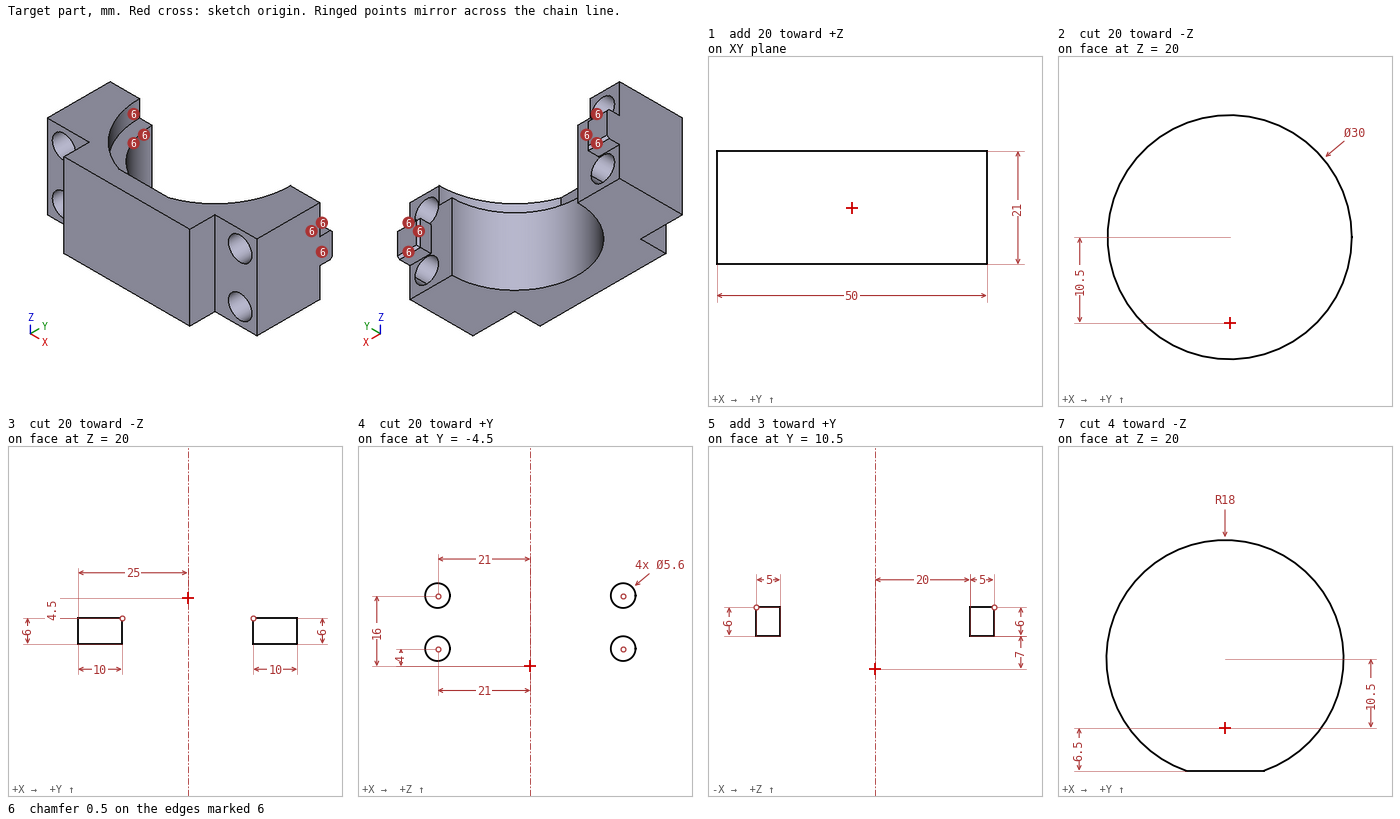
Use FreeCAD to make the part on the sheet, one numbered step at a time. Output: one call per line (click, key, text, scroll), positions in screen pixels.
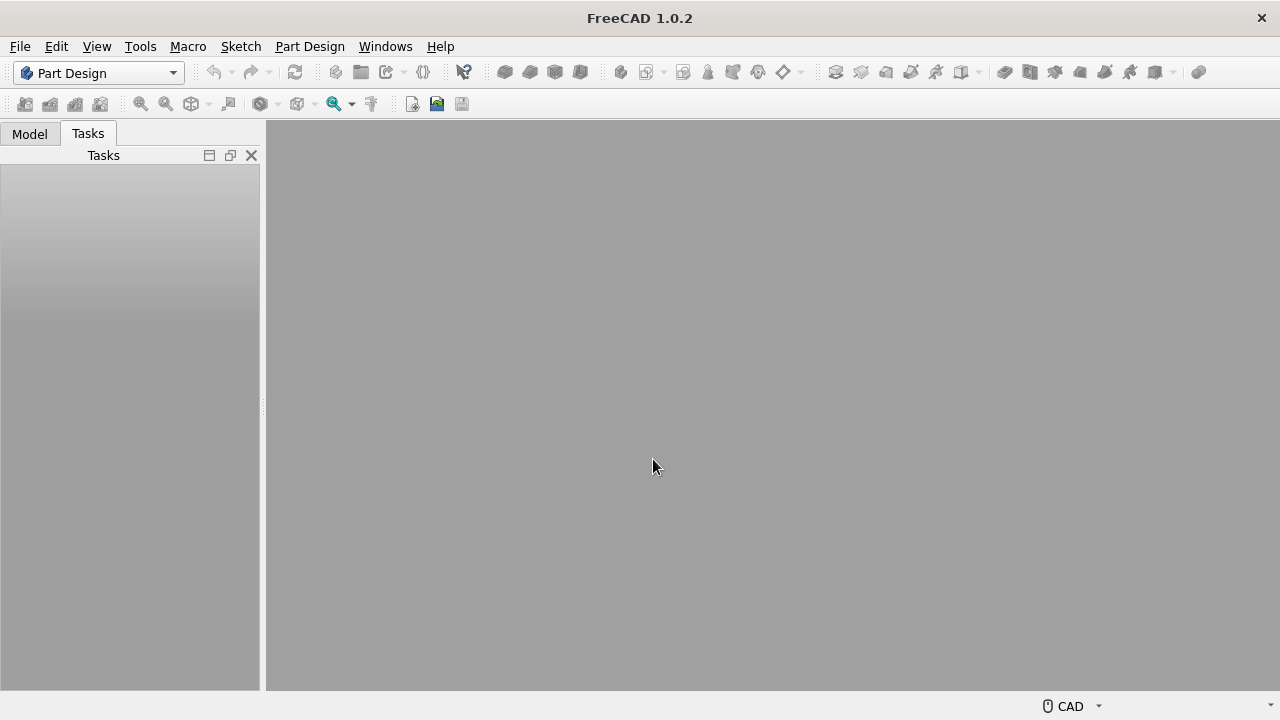
key(ctrl+n)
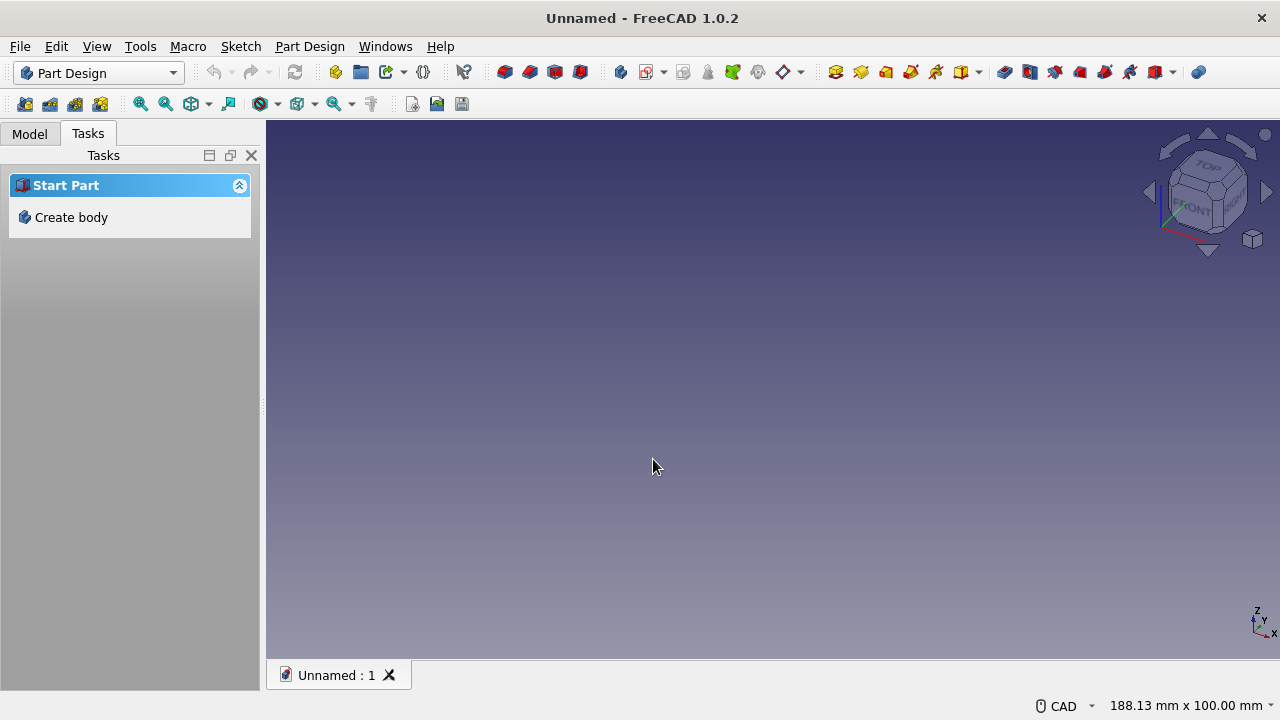
click(646, 72)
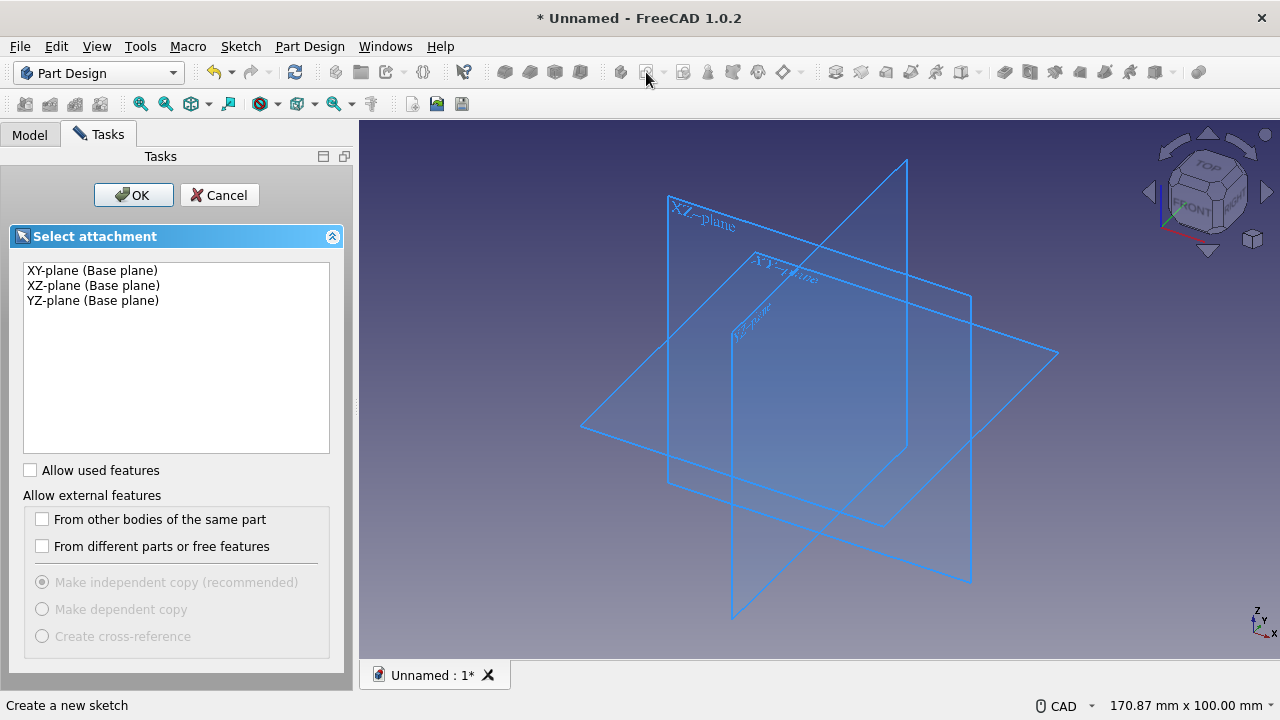
click(84, 270)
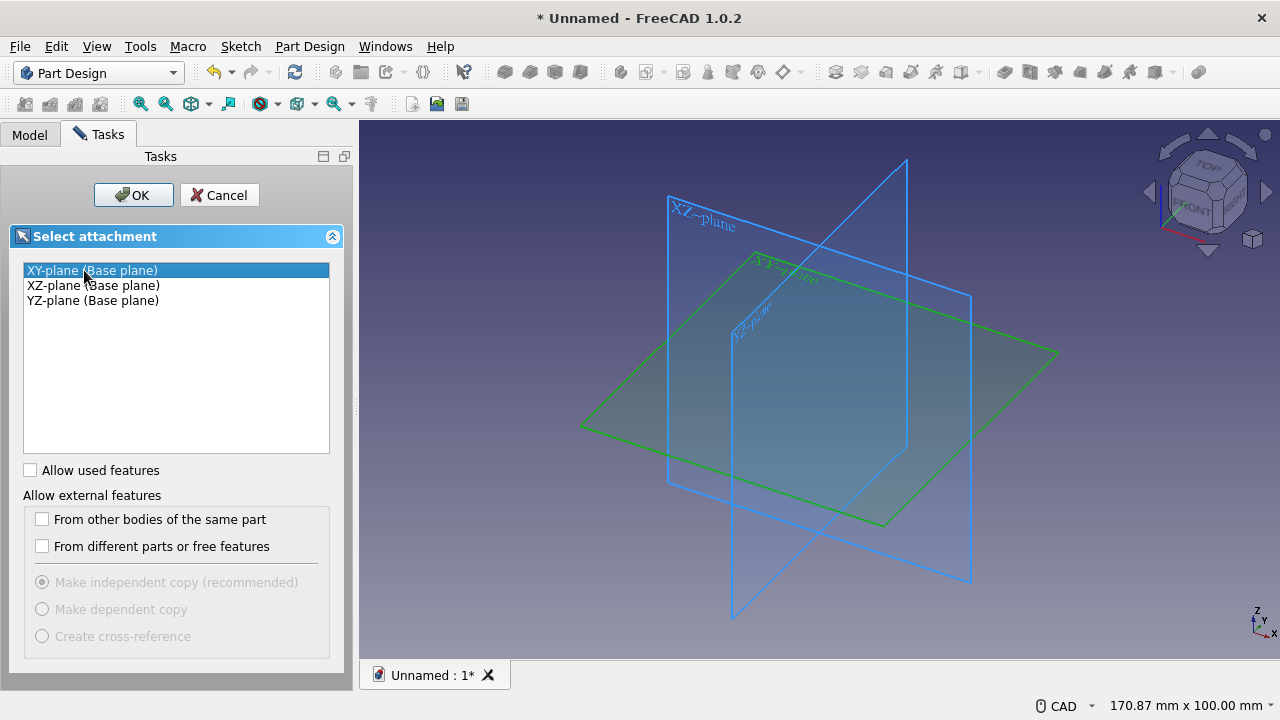
click(134, 195)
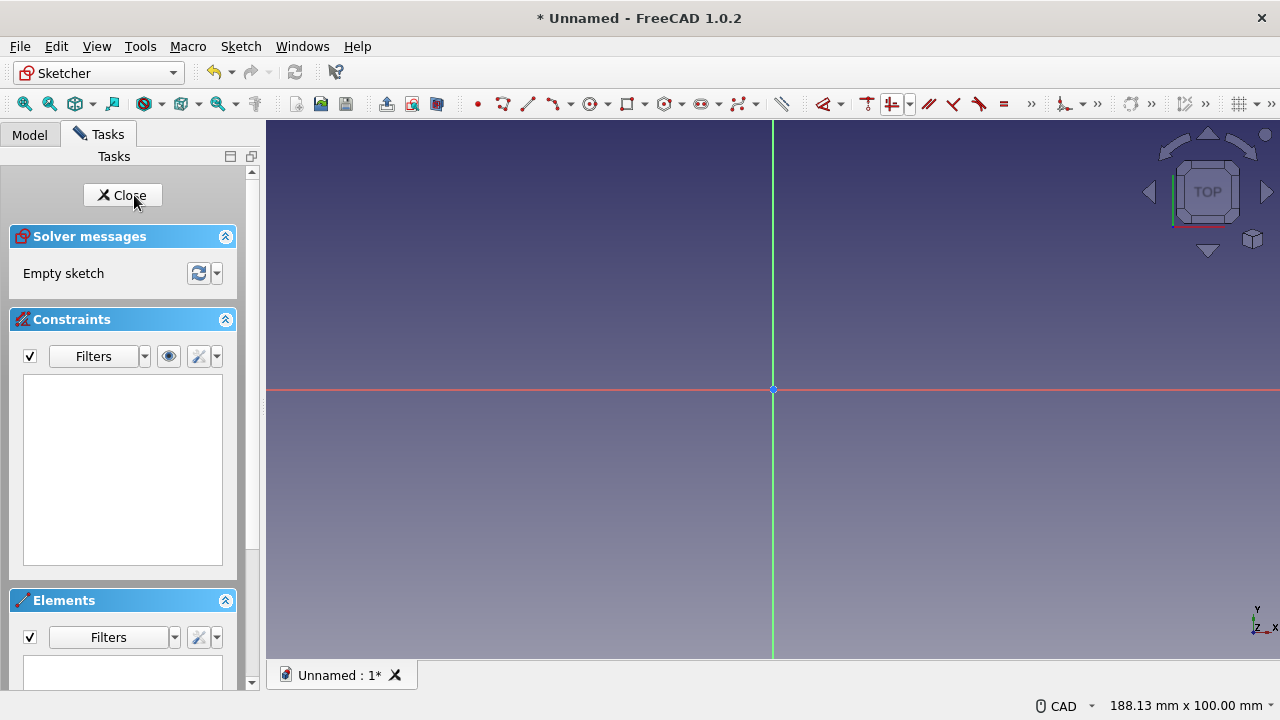
scroll(829, 390, up, 4)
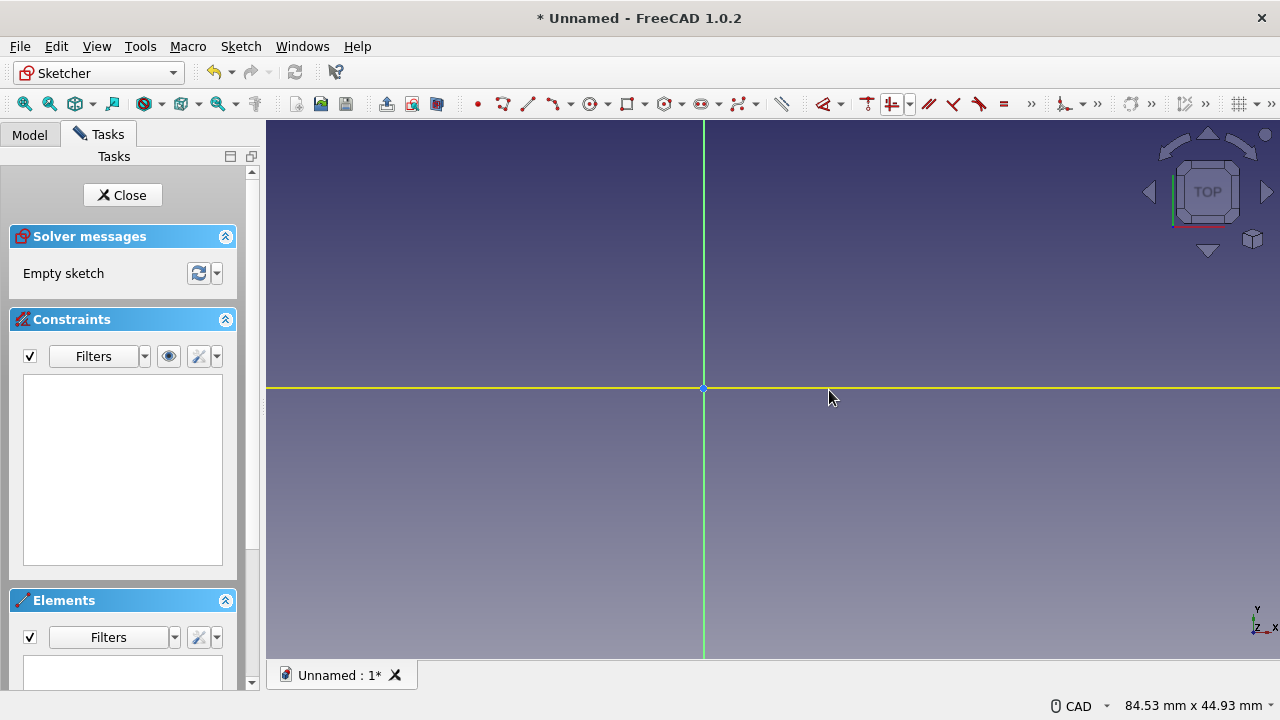
key(g)
key(v)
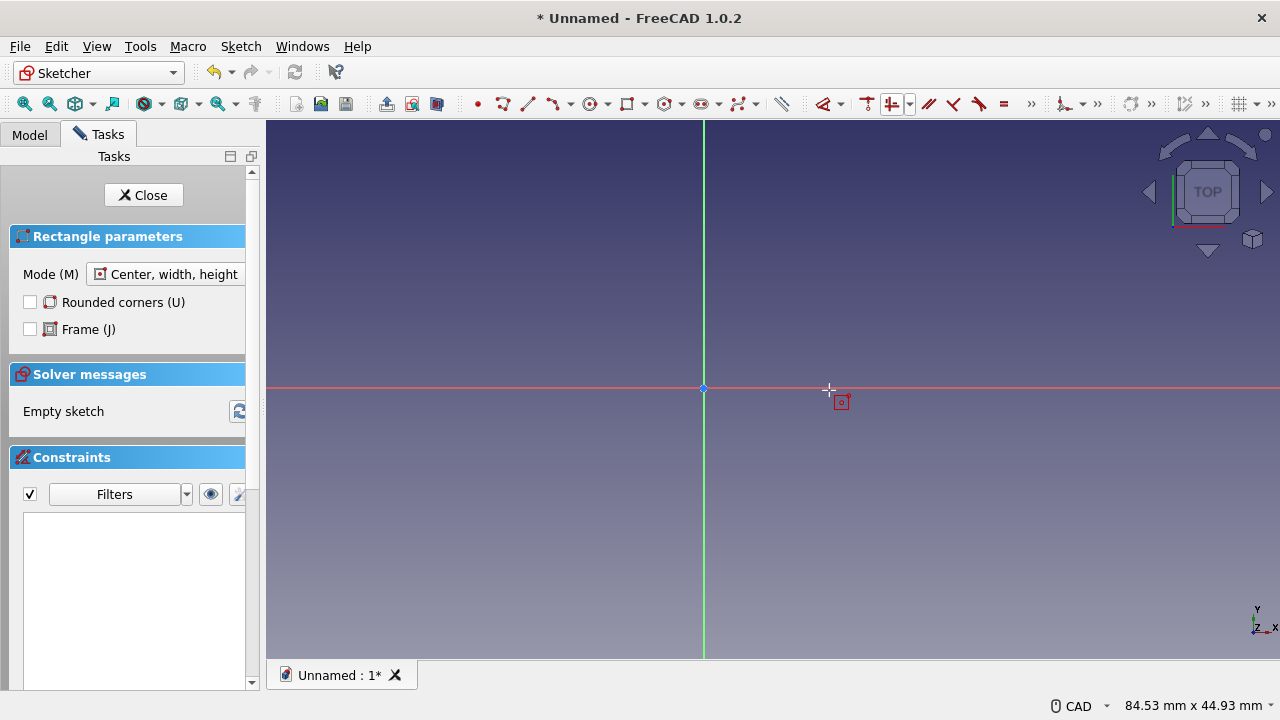
click(704, 388)
move(1004, 262)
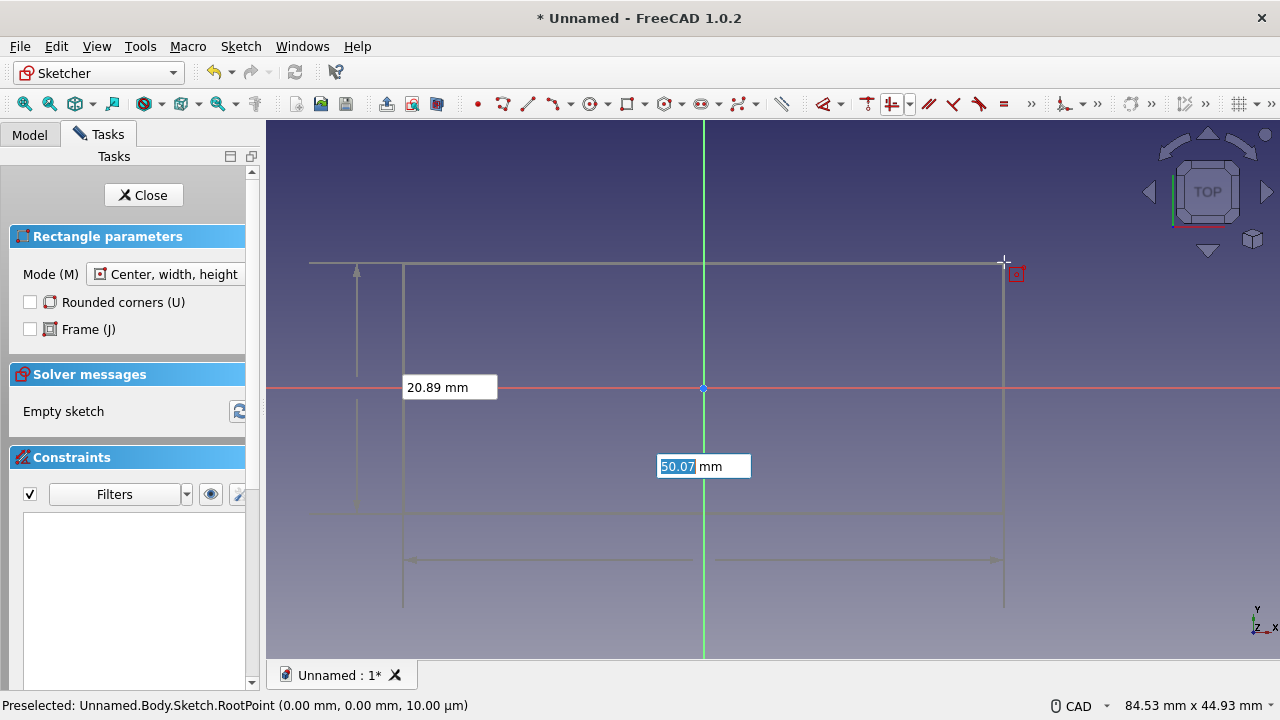
text(50)
key(Tab)
text(21)
key(Return)
key(Escape)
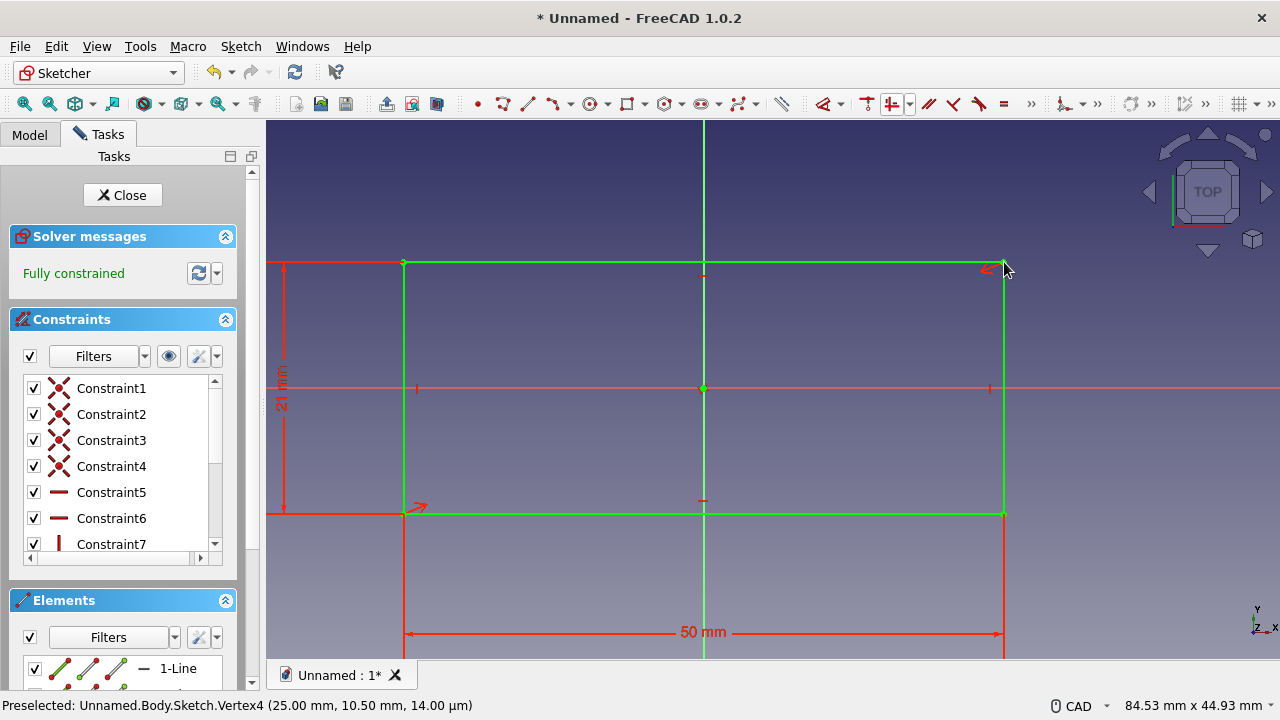
click(123, 195)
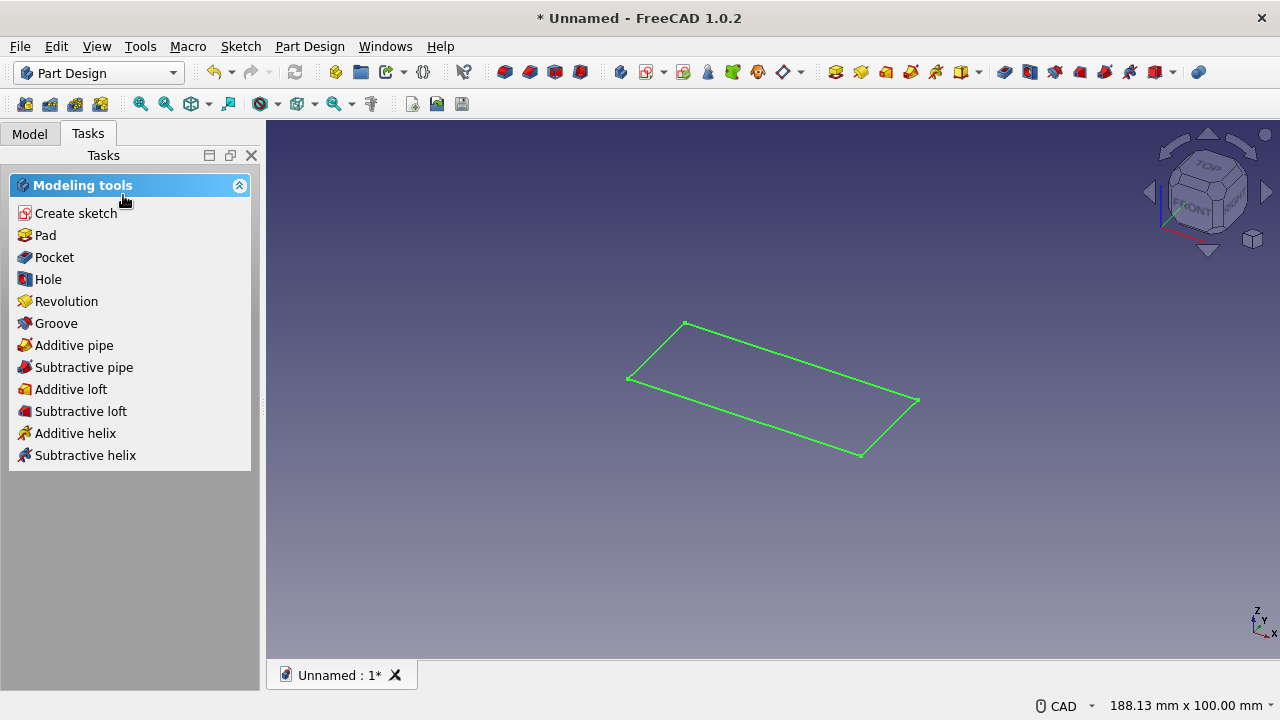
click(836, 72)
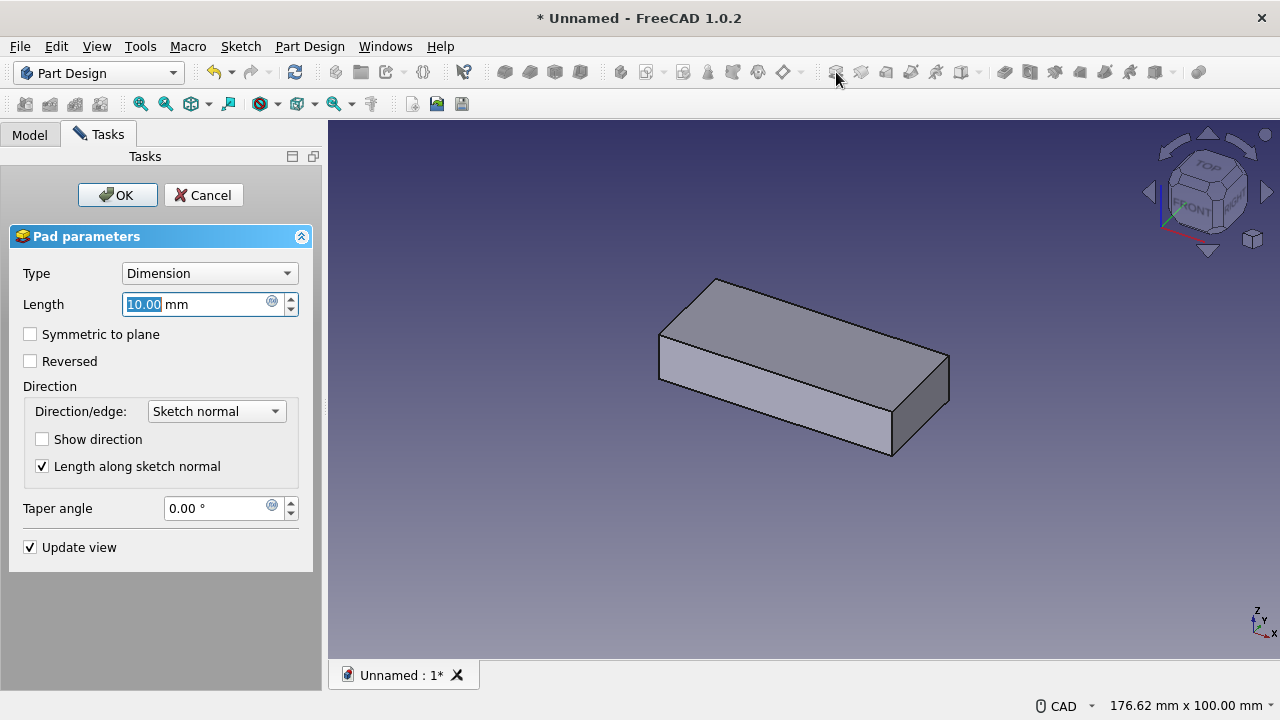
text(20)
key(Tab)